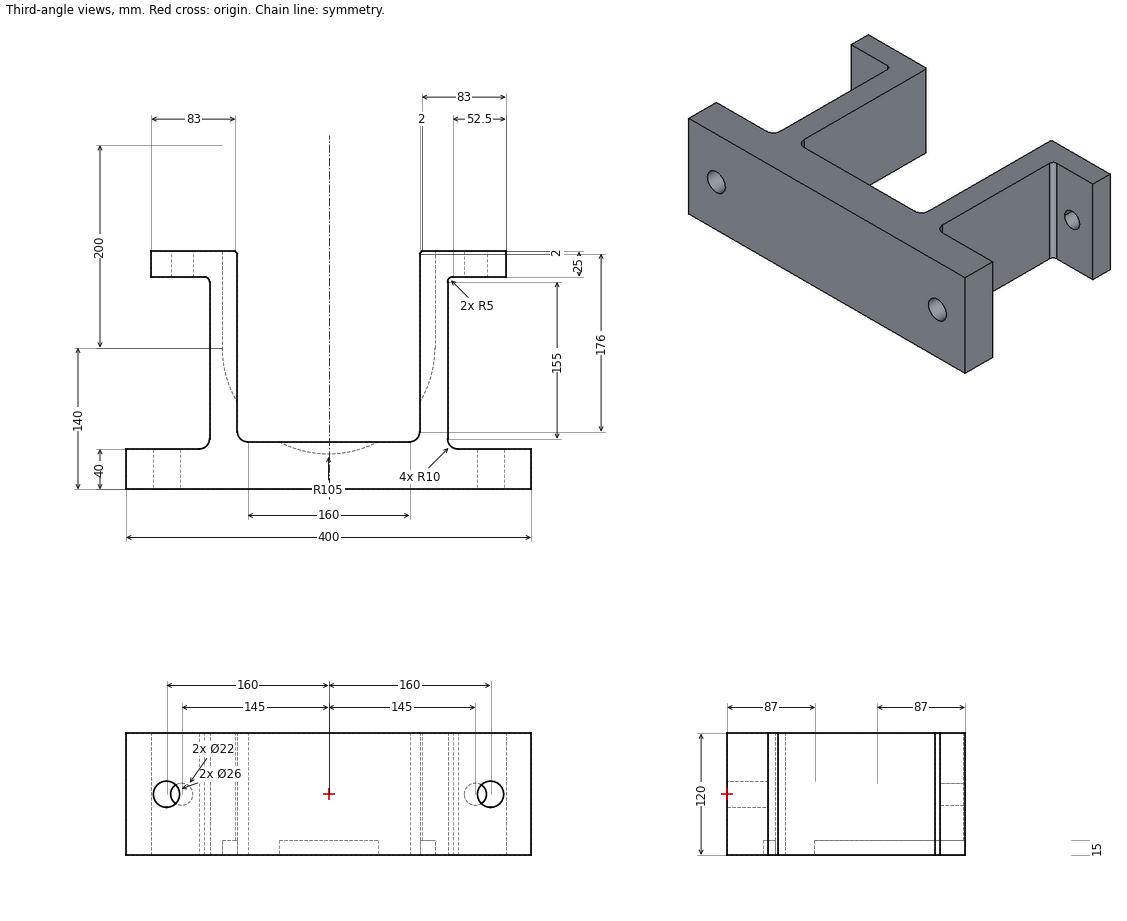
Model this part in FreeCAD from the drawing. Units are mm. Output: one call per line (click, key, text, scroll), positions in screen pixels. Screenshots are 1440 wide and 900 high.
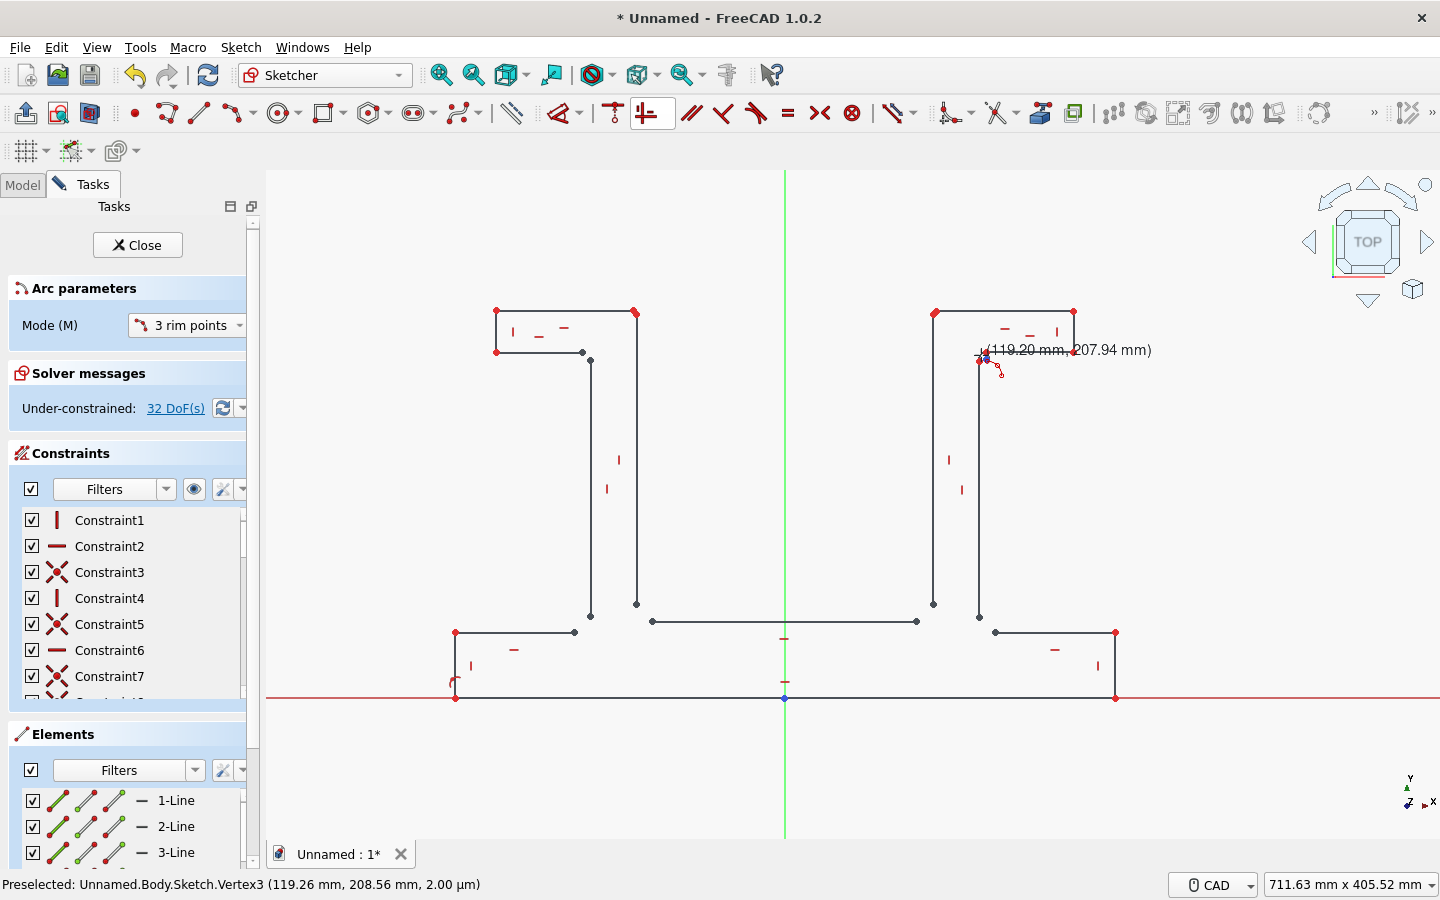
click(933, 605)
click(917, 622)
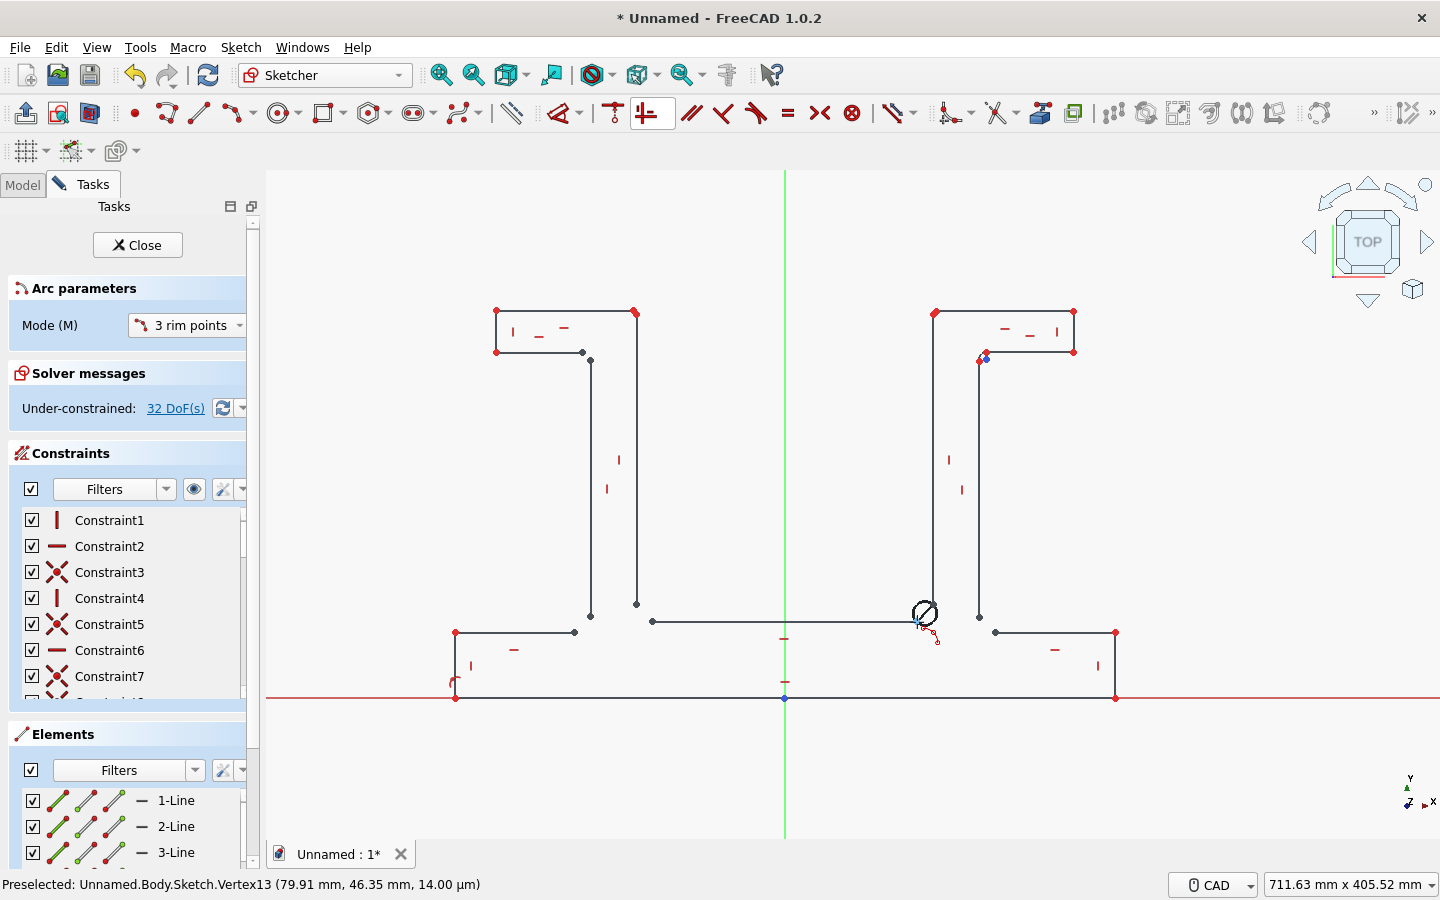
scroll(929, 616, up, 6)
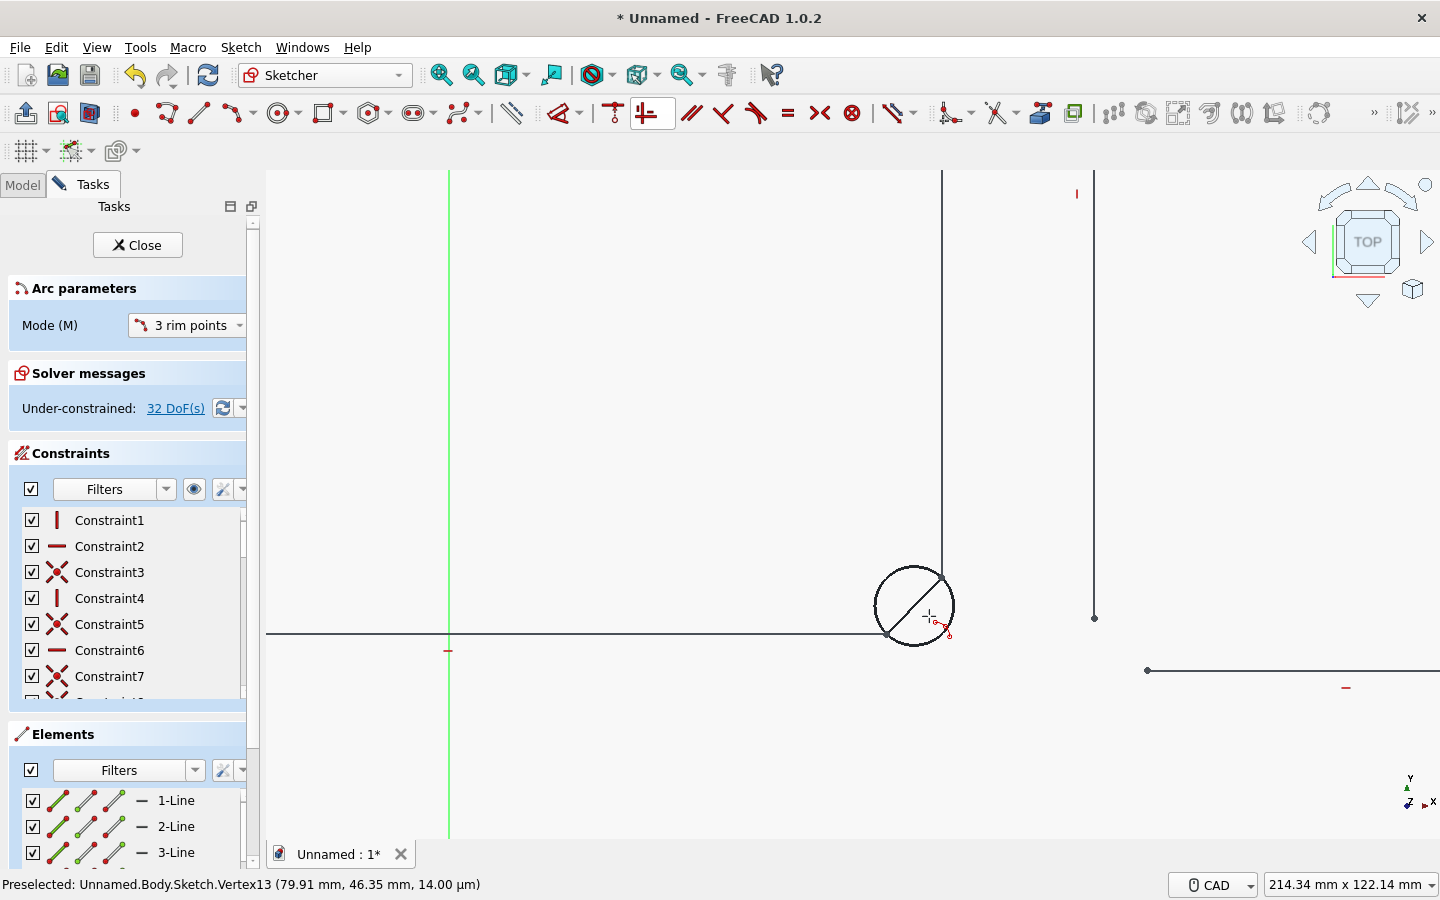
click(926, 615)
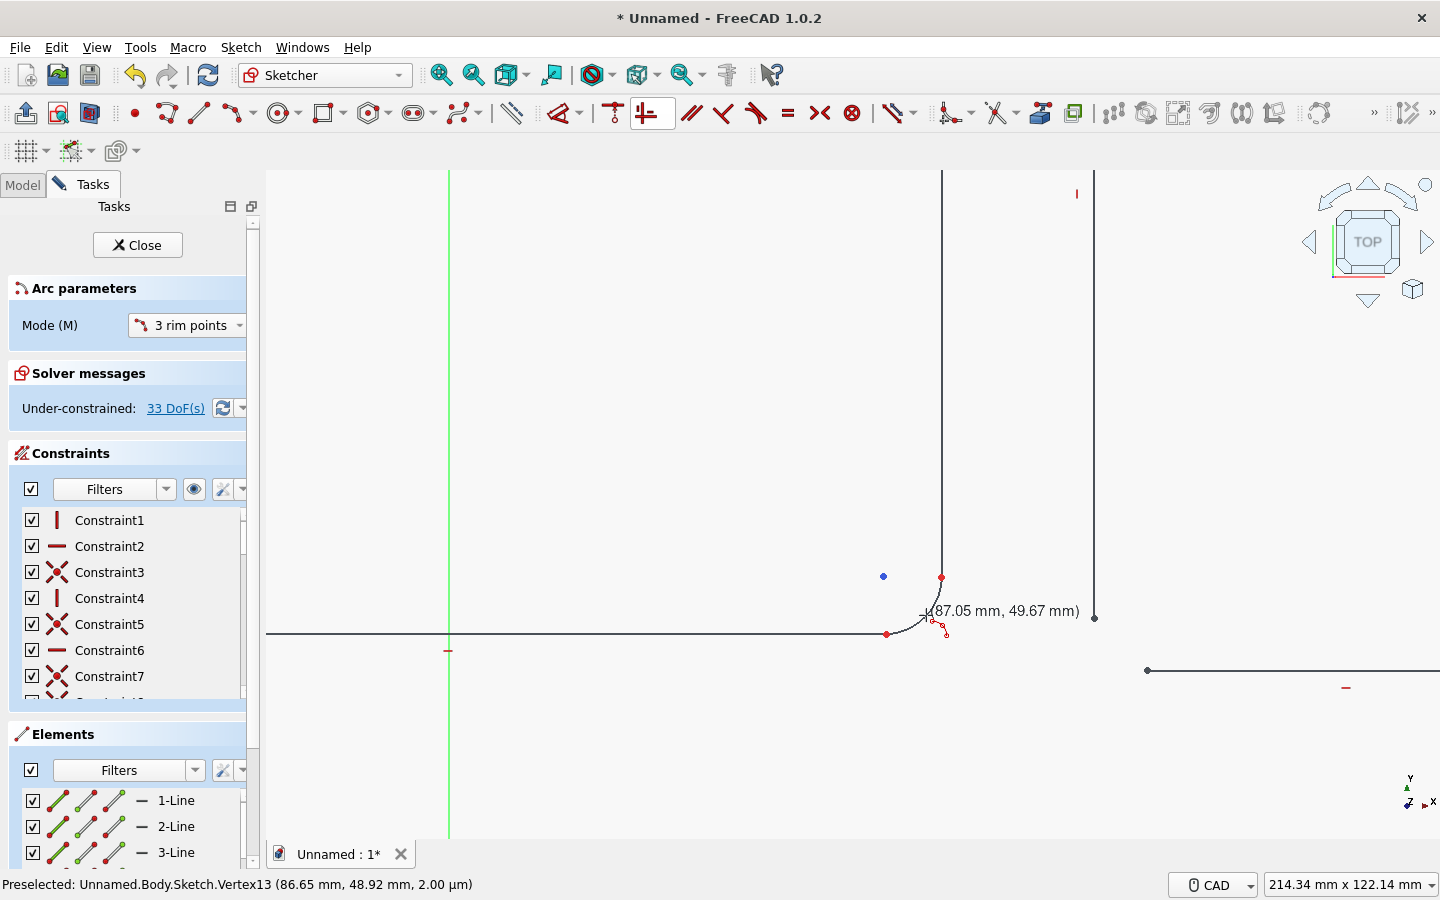
scroll(929, 617, down, 6)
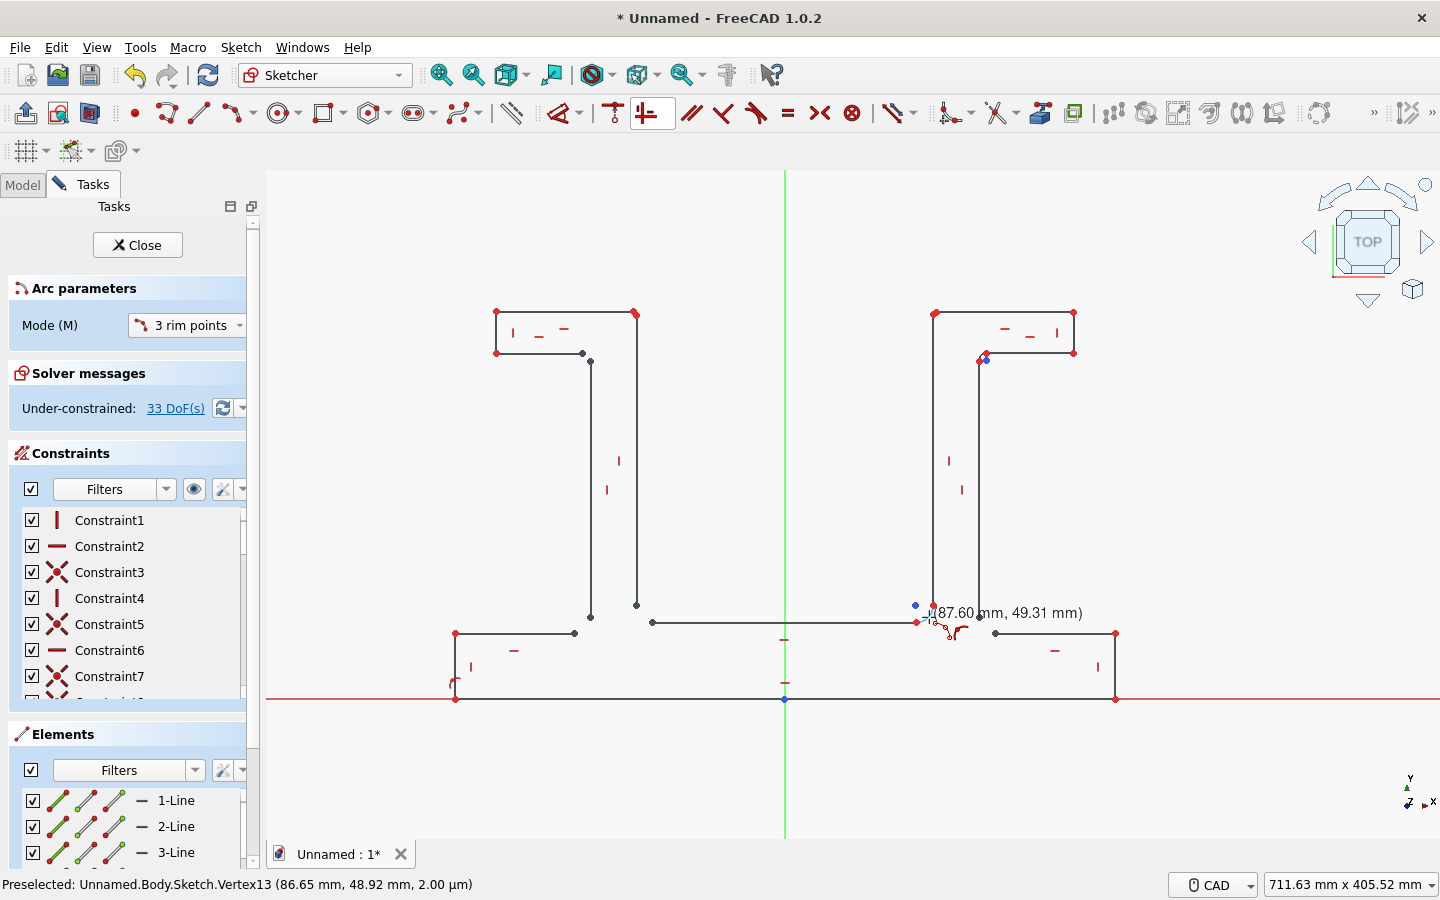
click(653, 623)
click(637, 606)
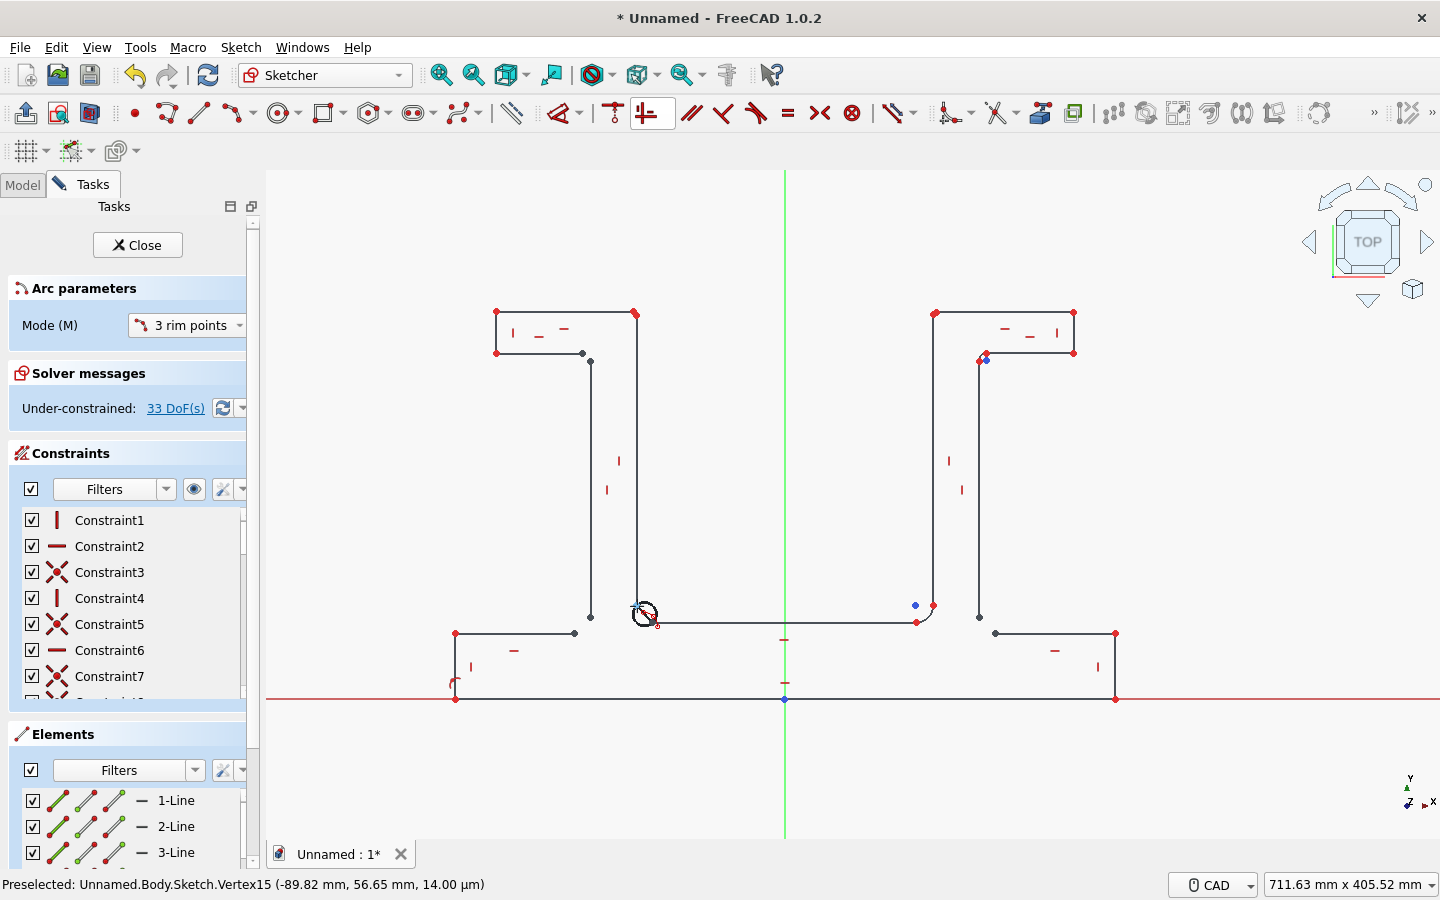
scroll(641, 617, up, 6)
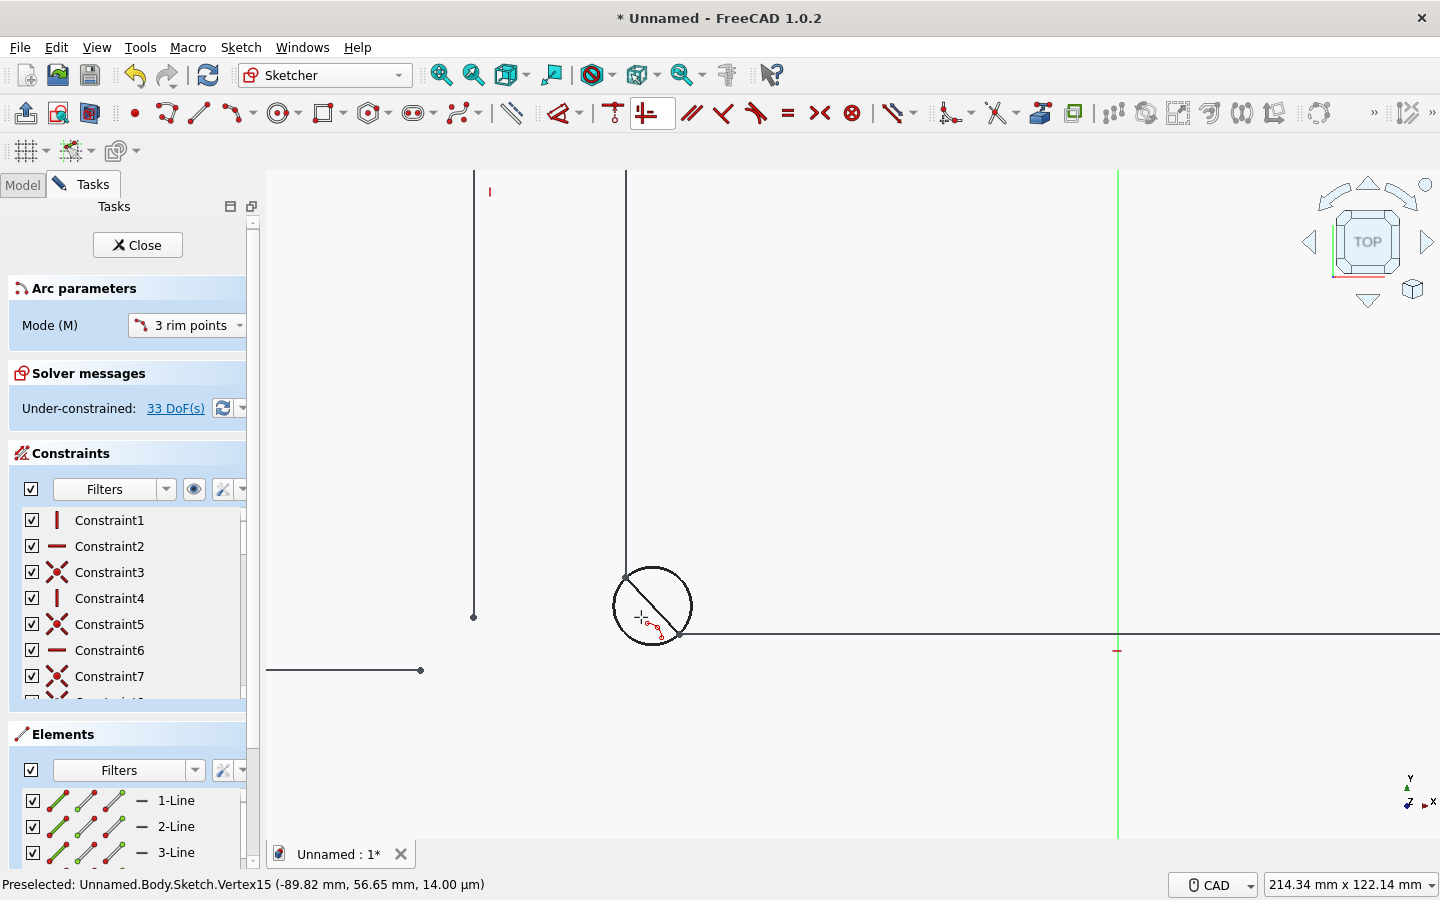
click(641, 615)